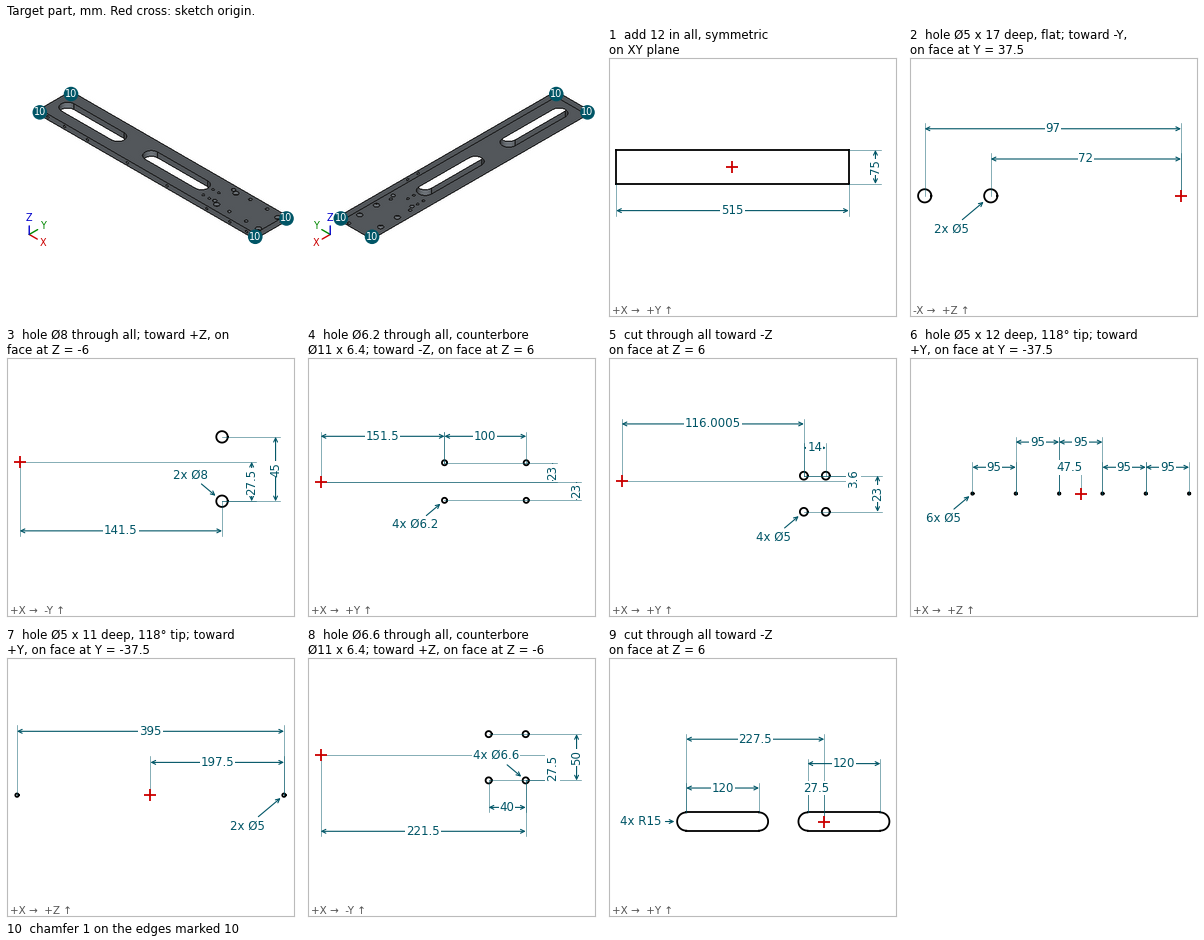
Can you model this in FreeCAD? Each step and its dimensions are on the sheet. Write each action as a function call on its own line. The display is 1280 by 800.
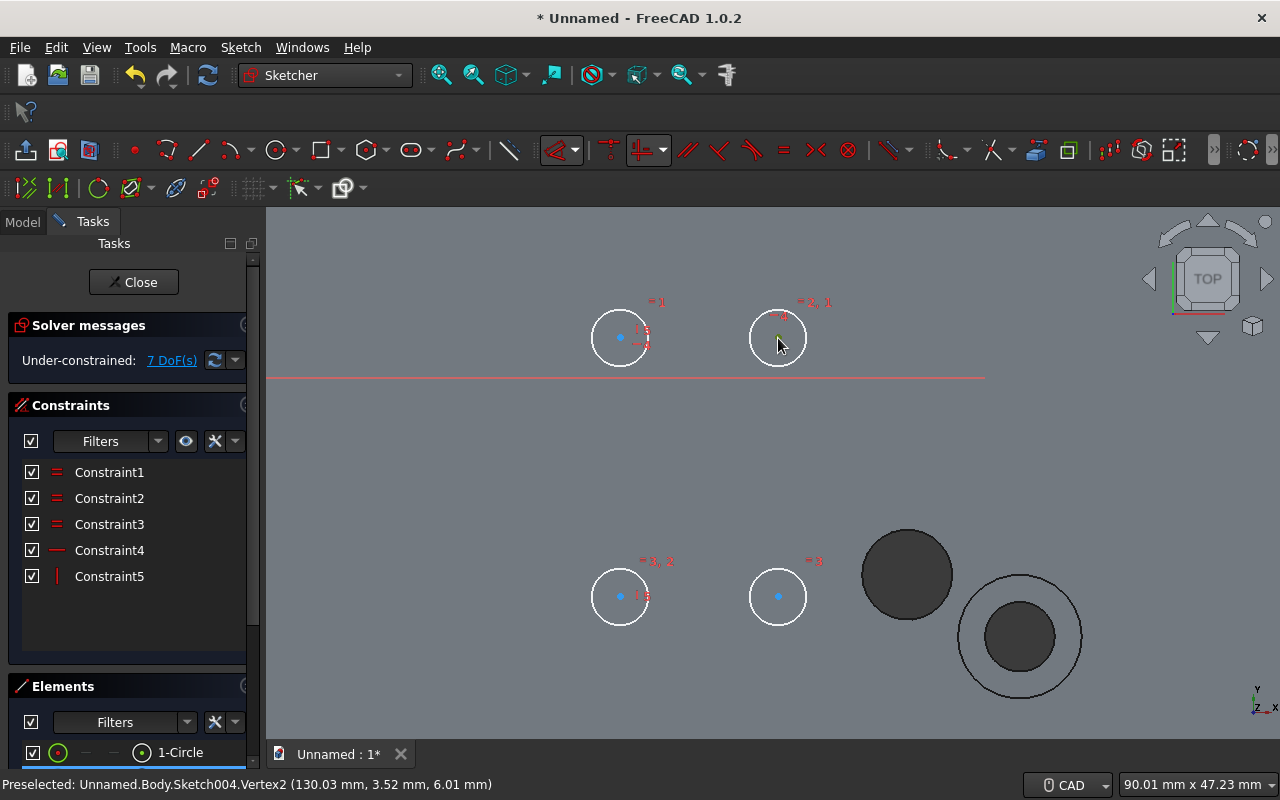
click(778, 597)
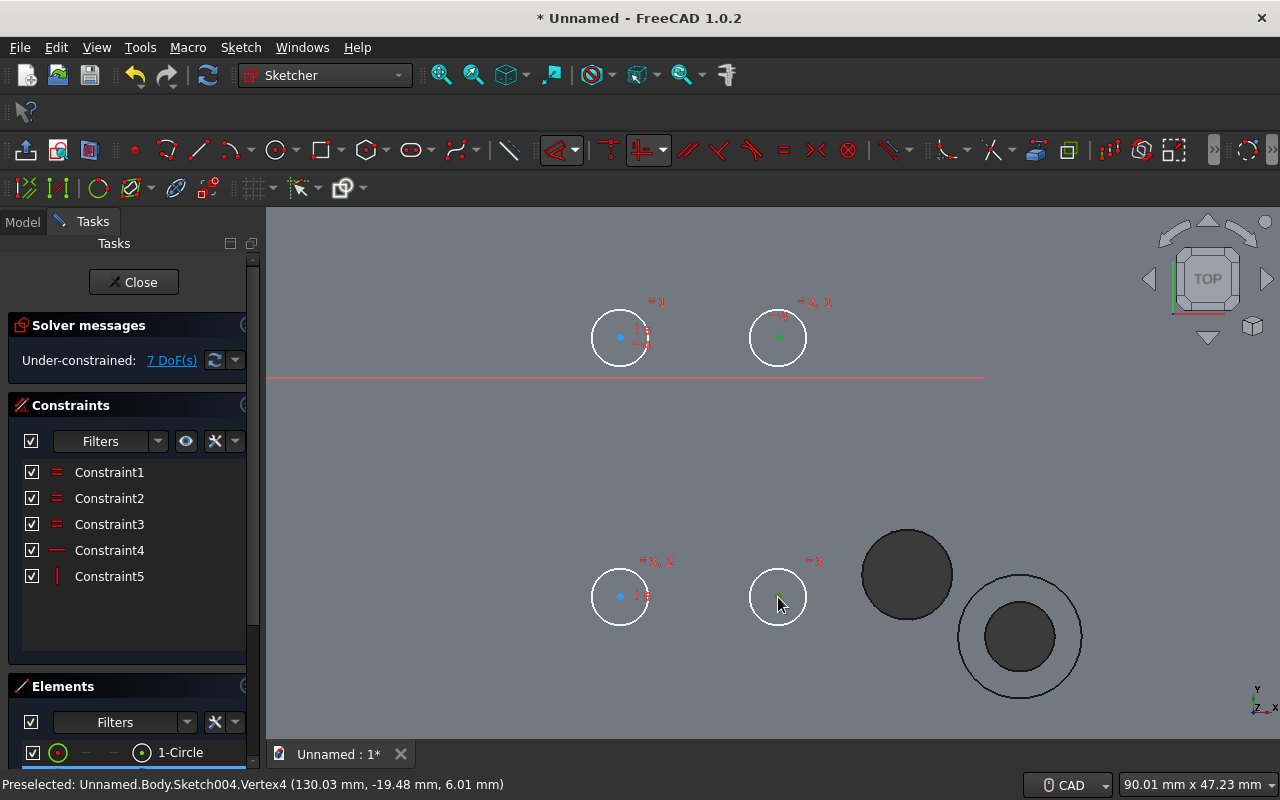
key(v)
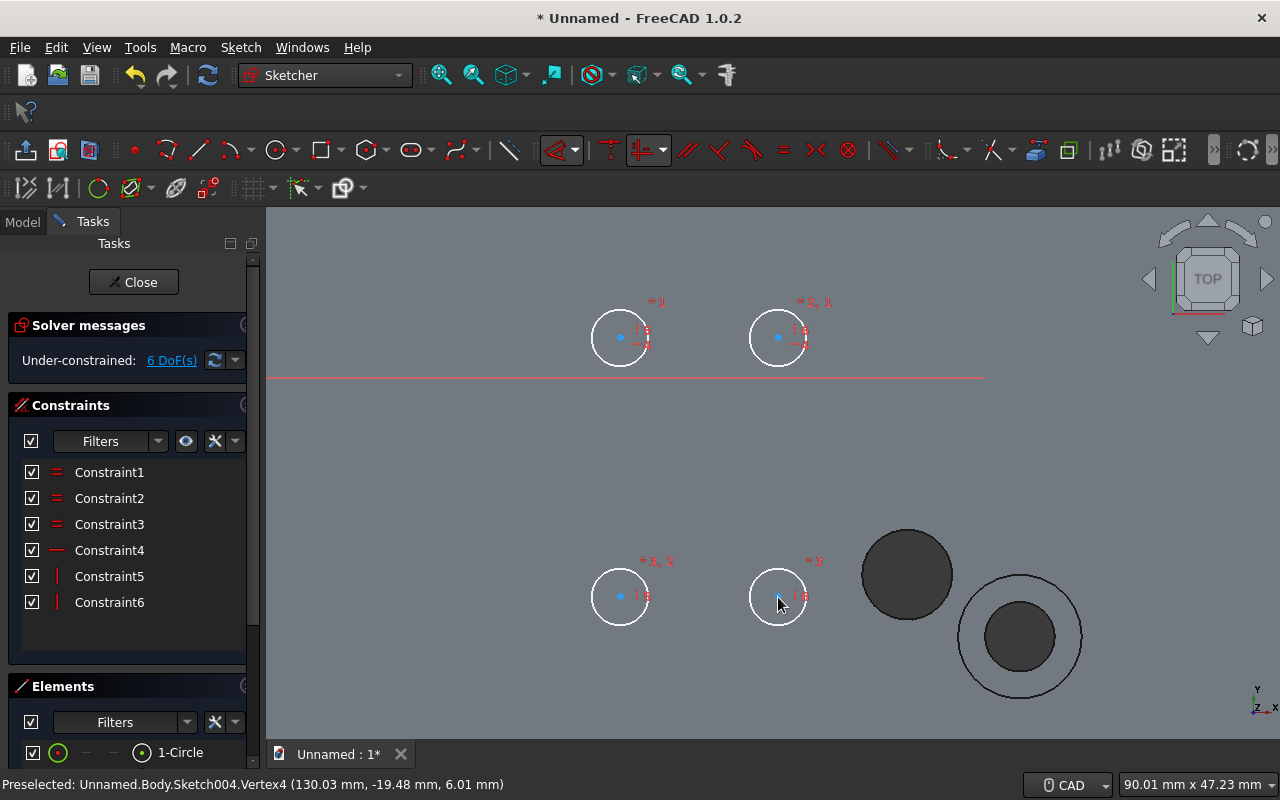
click(620, 597)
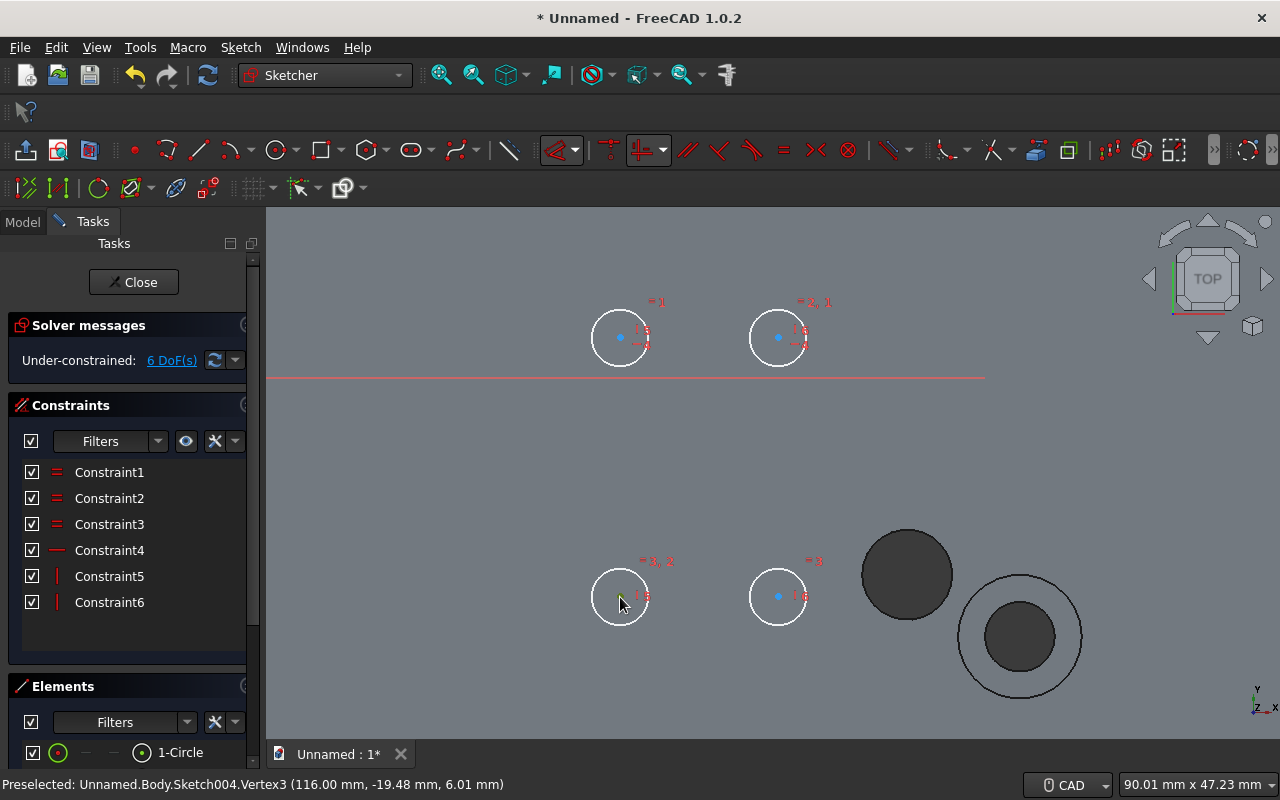
click(778, 597)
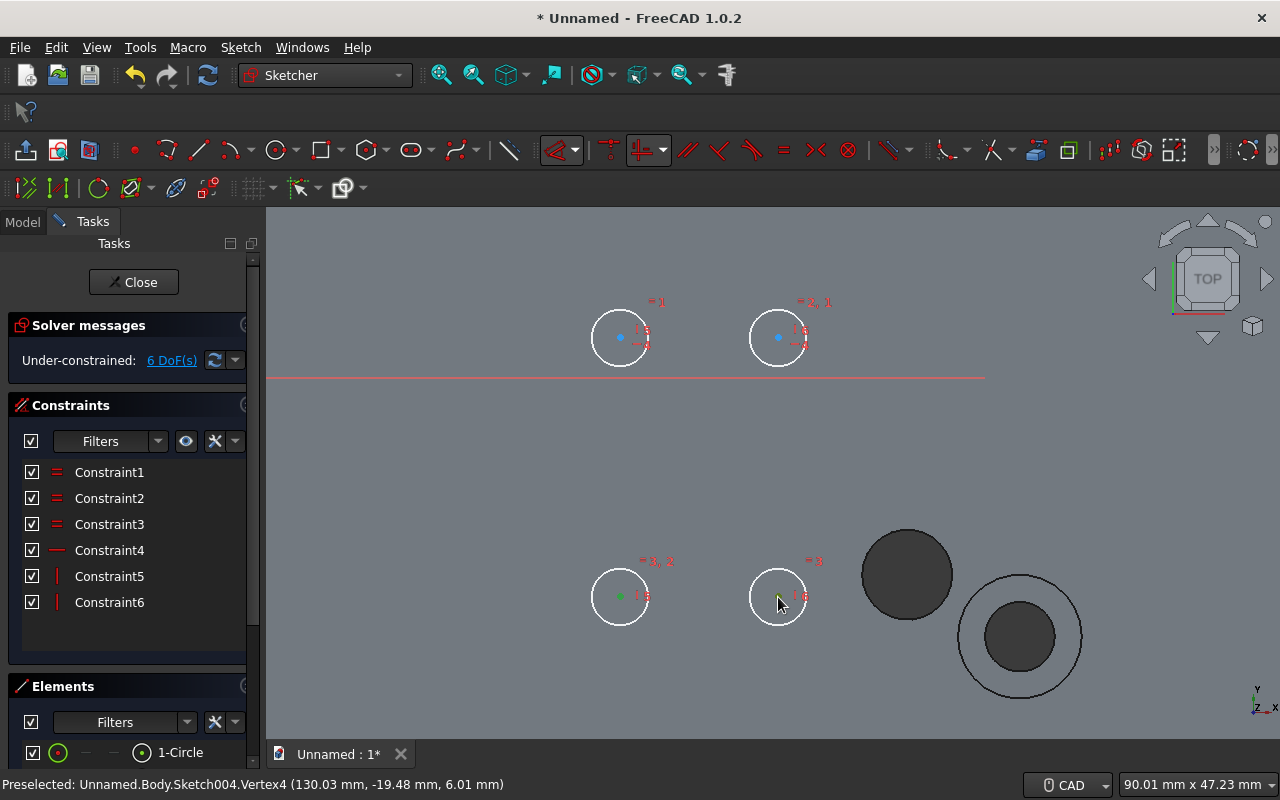
key(h)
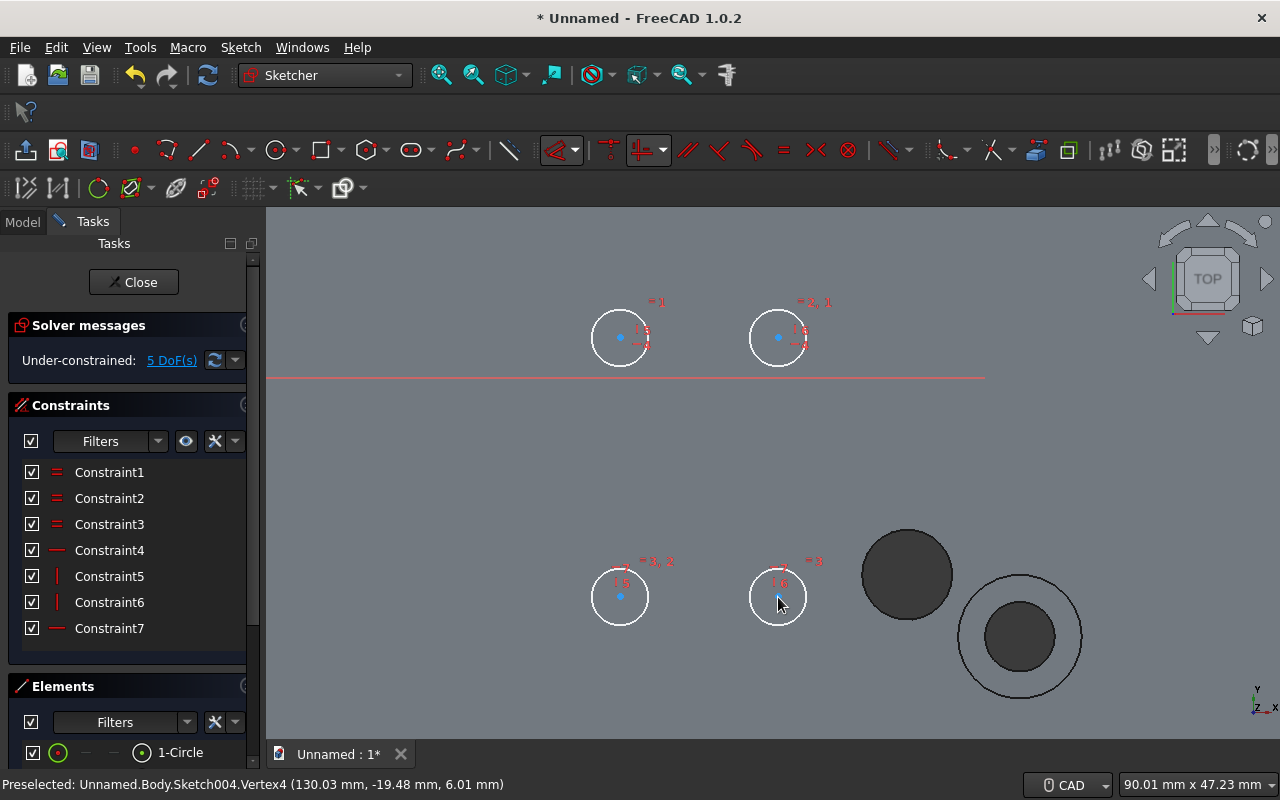
click(556, 150)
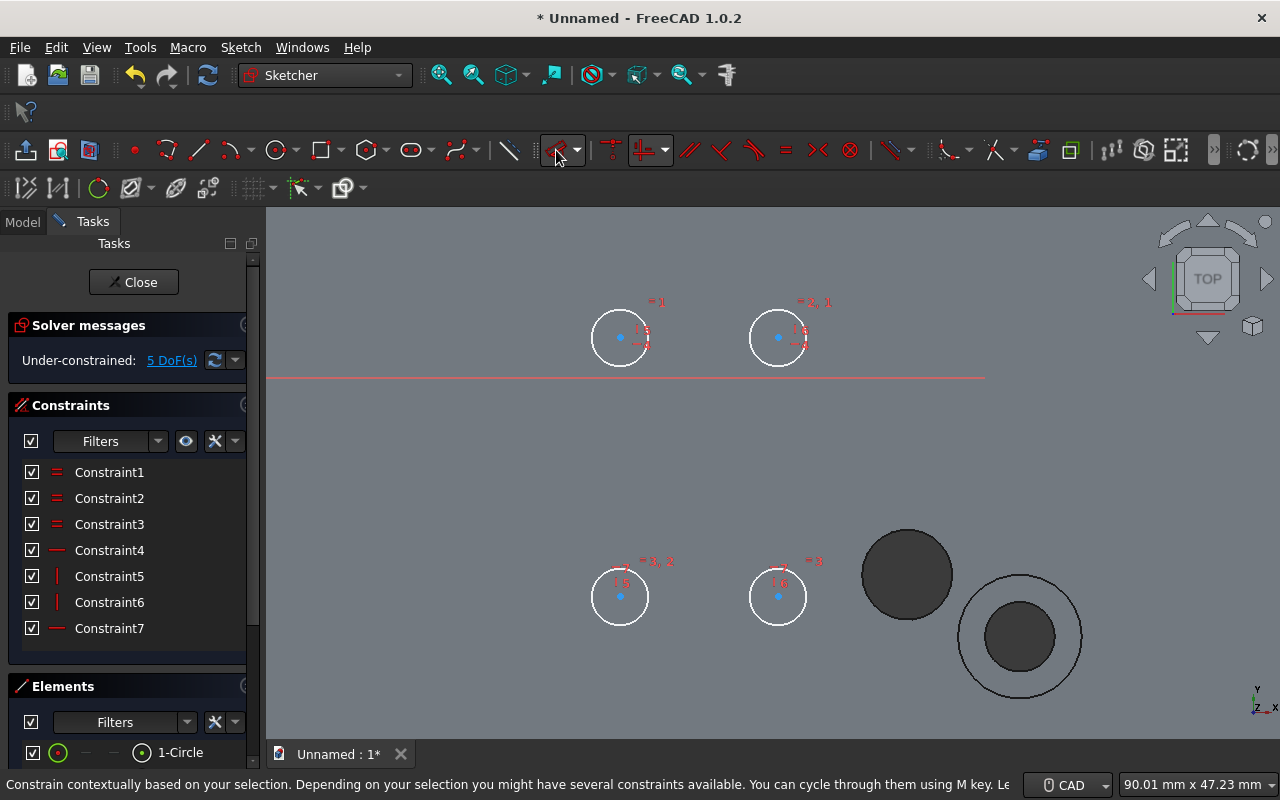
click(640, 318)
click(663, 295)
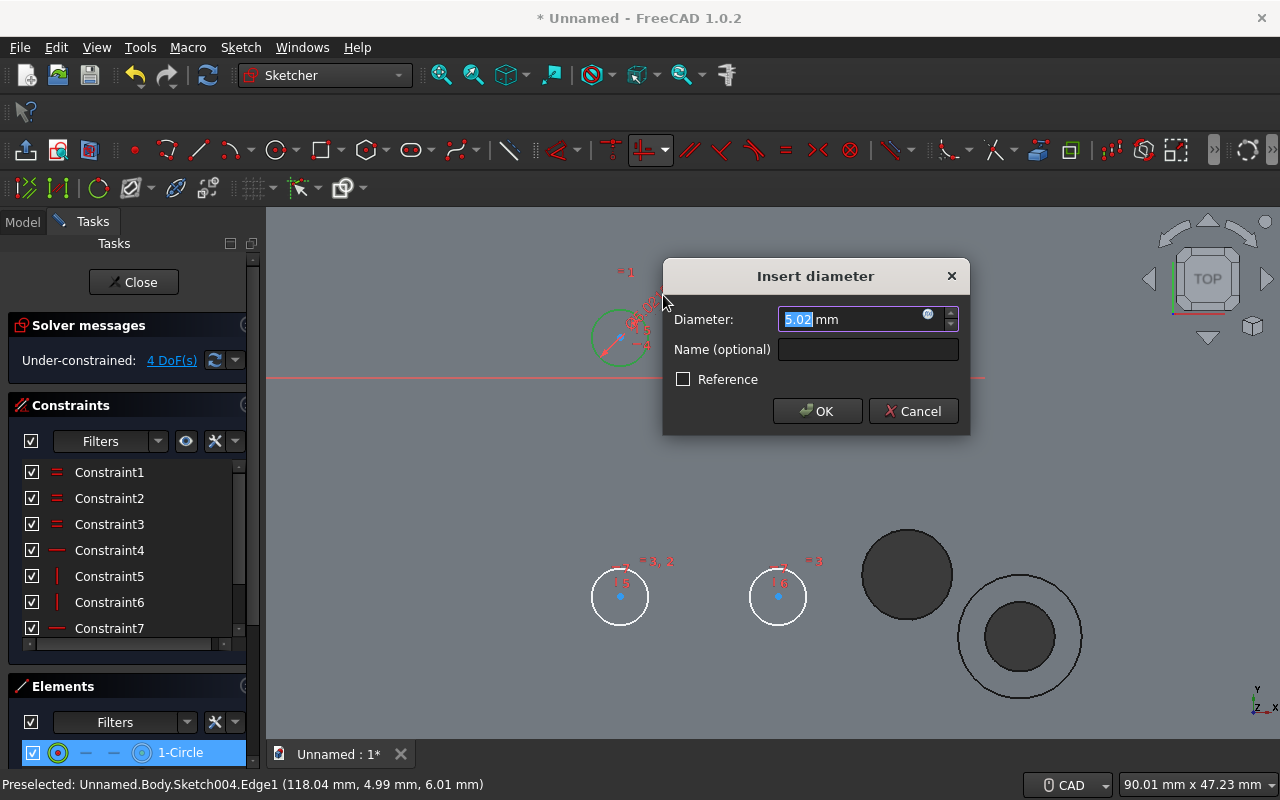
text(5)
key(Return)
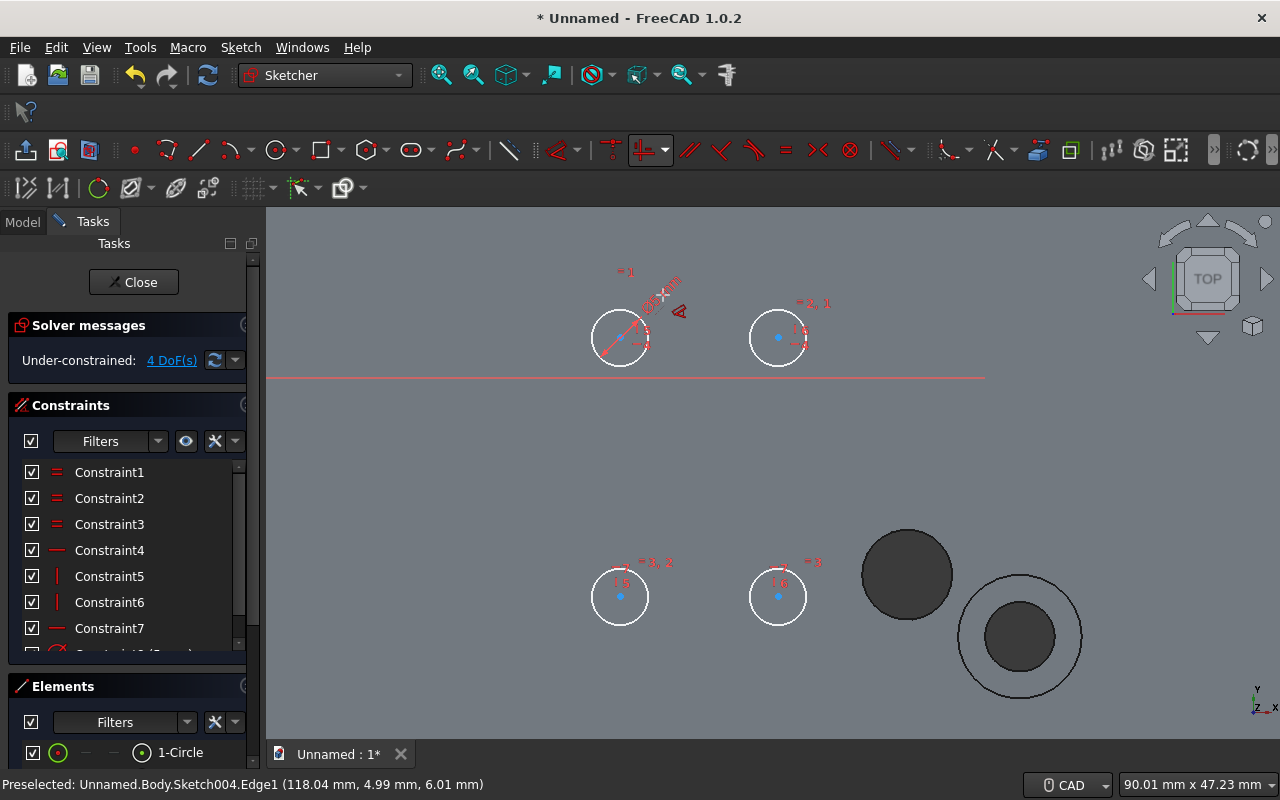
click(620, 338)
click(678, 358)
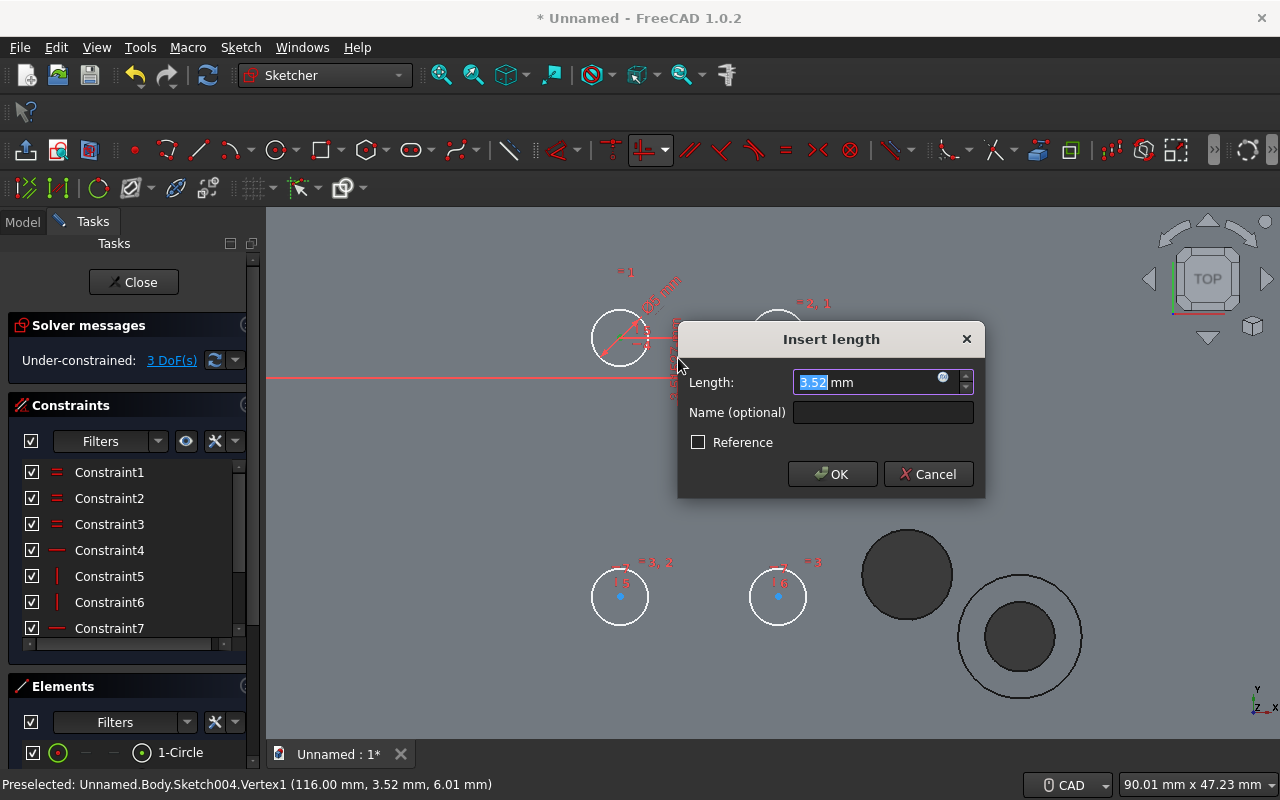
text(3.6)
key(Return)